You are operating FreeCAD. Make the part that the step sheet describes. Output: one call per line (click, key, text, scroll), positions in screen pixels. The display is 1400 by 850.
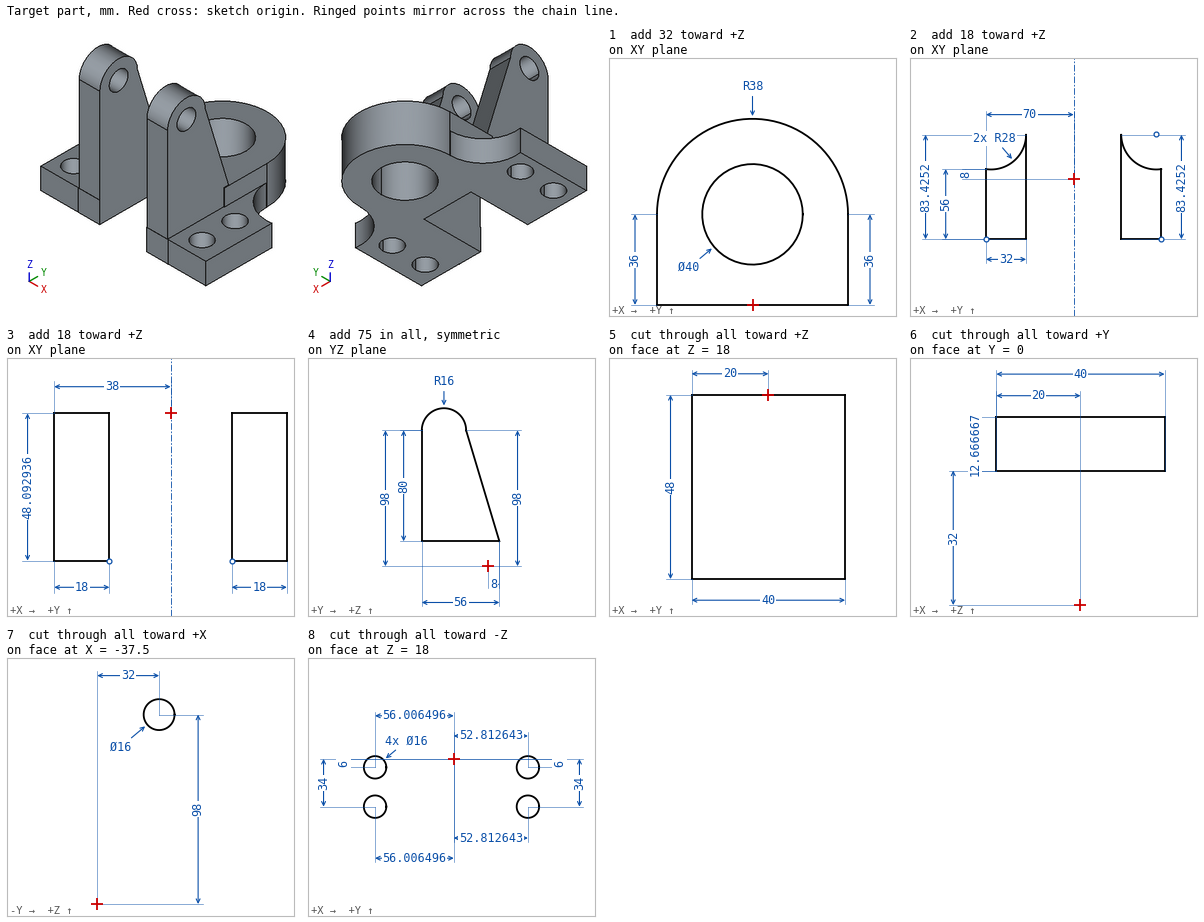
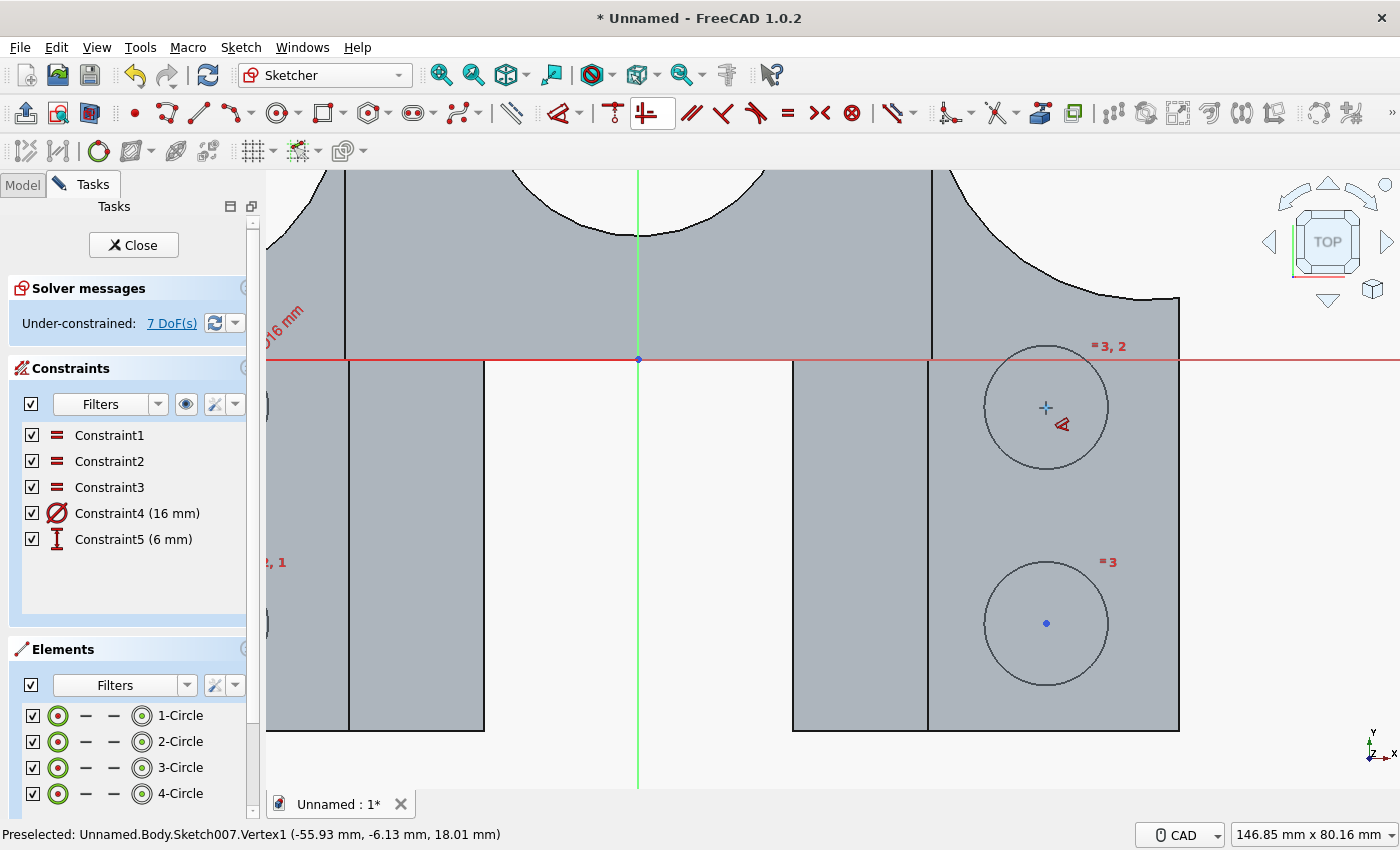
click(1046, 407)
click(1080, 384)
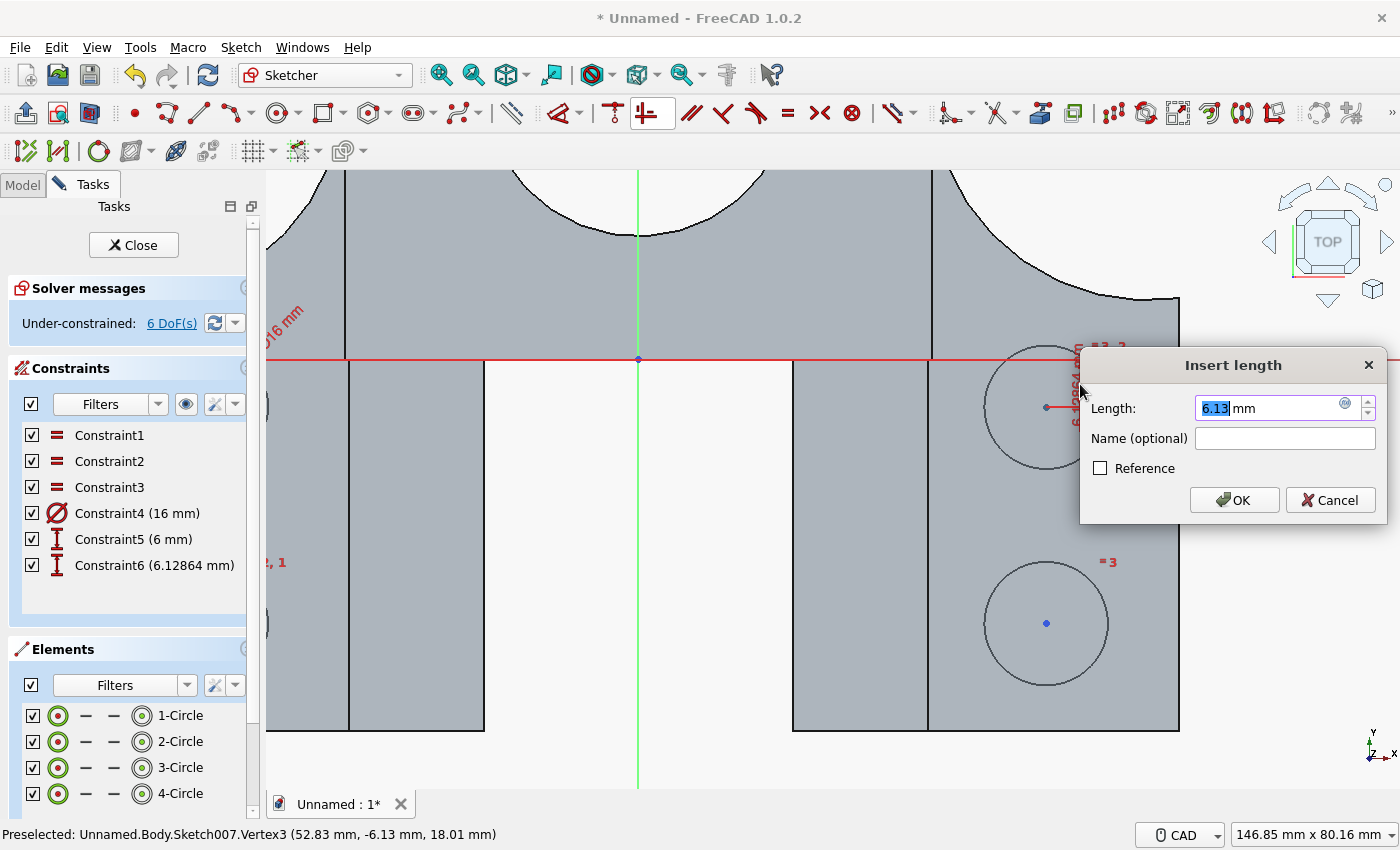
text(6)
key(Return)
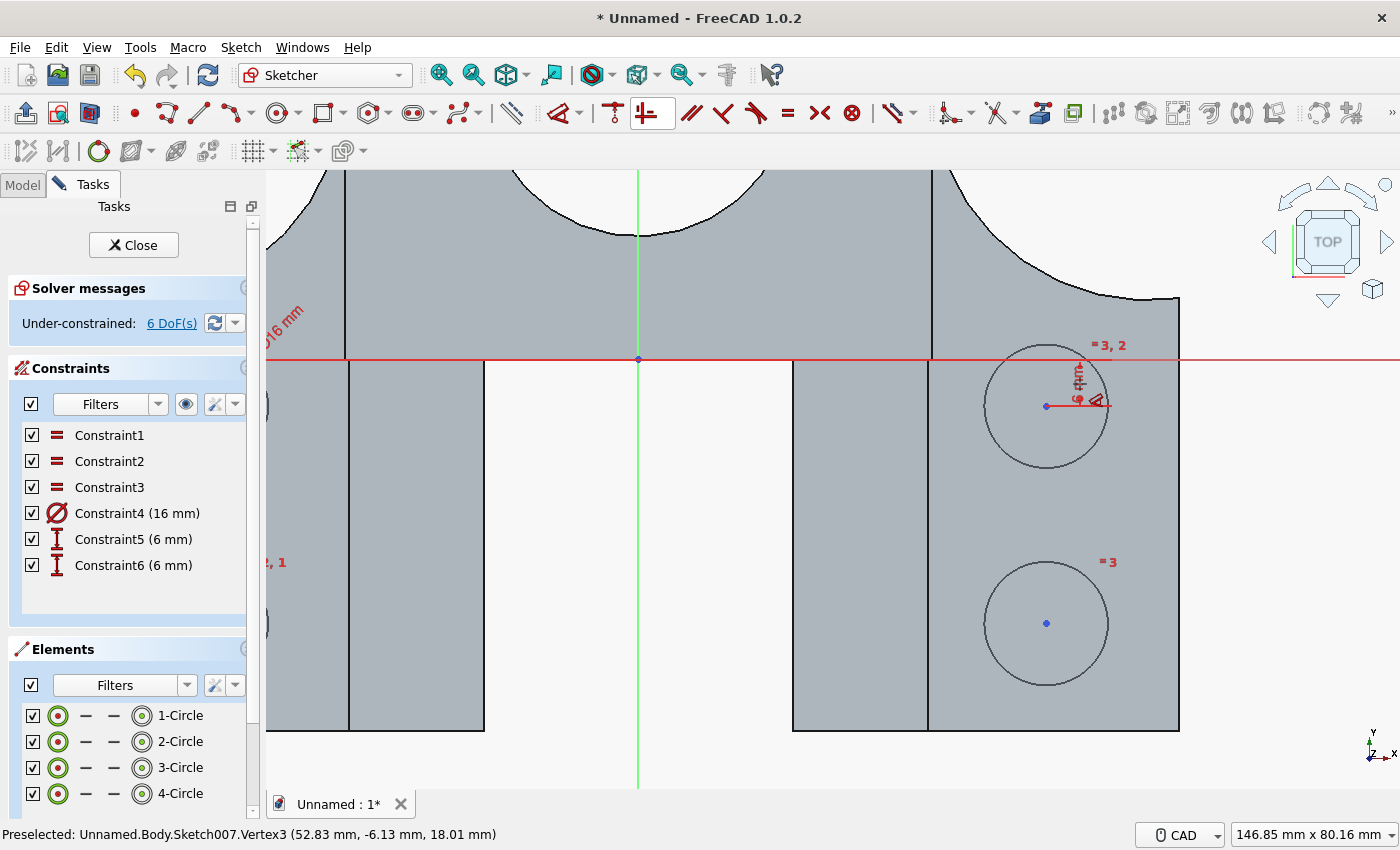
scroll(1046, 408, down, 2)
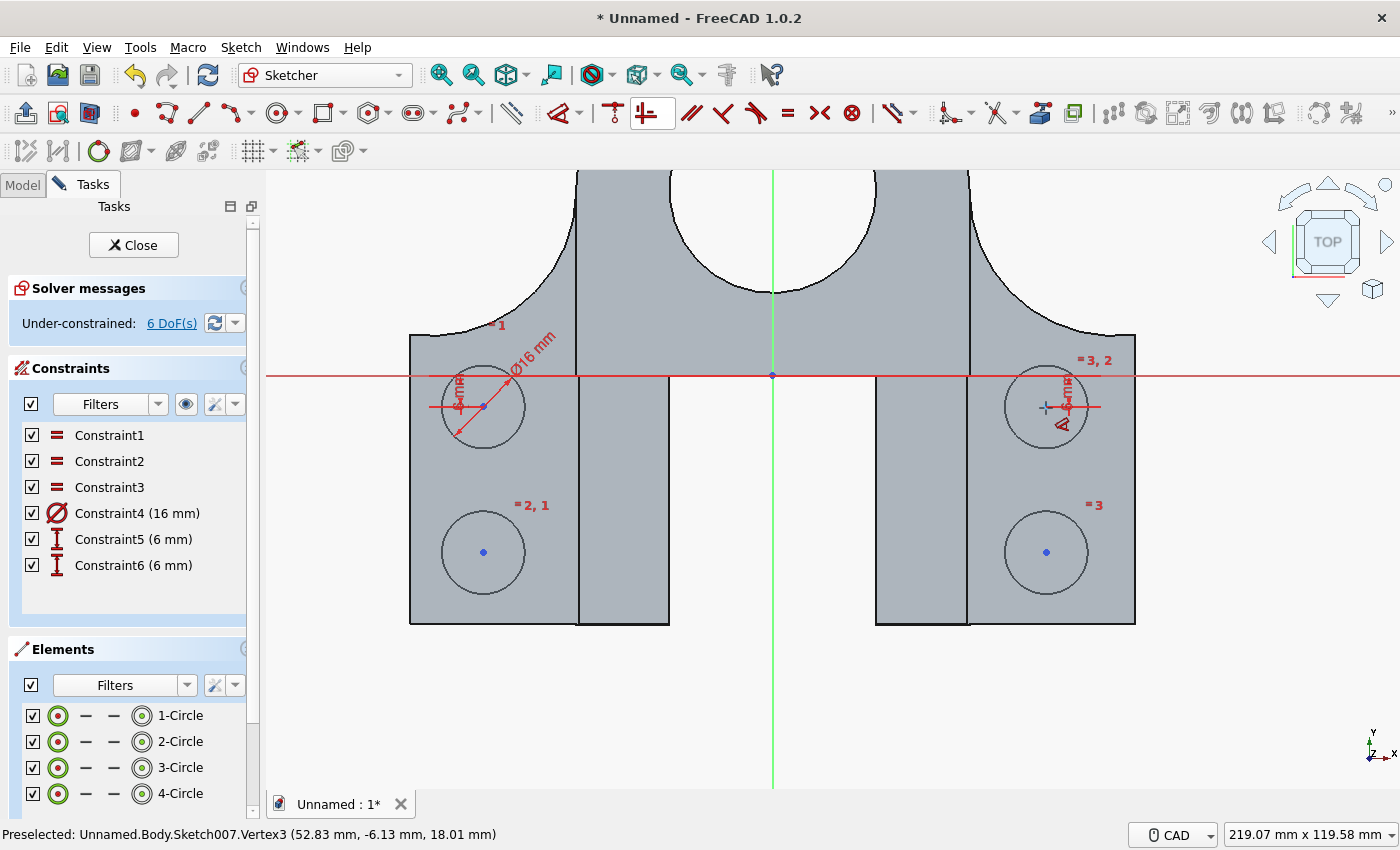
click(483, 553)
click(449, 464)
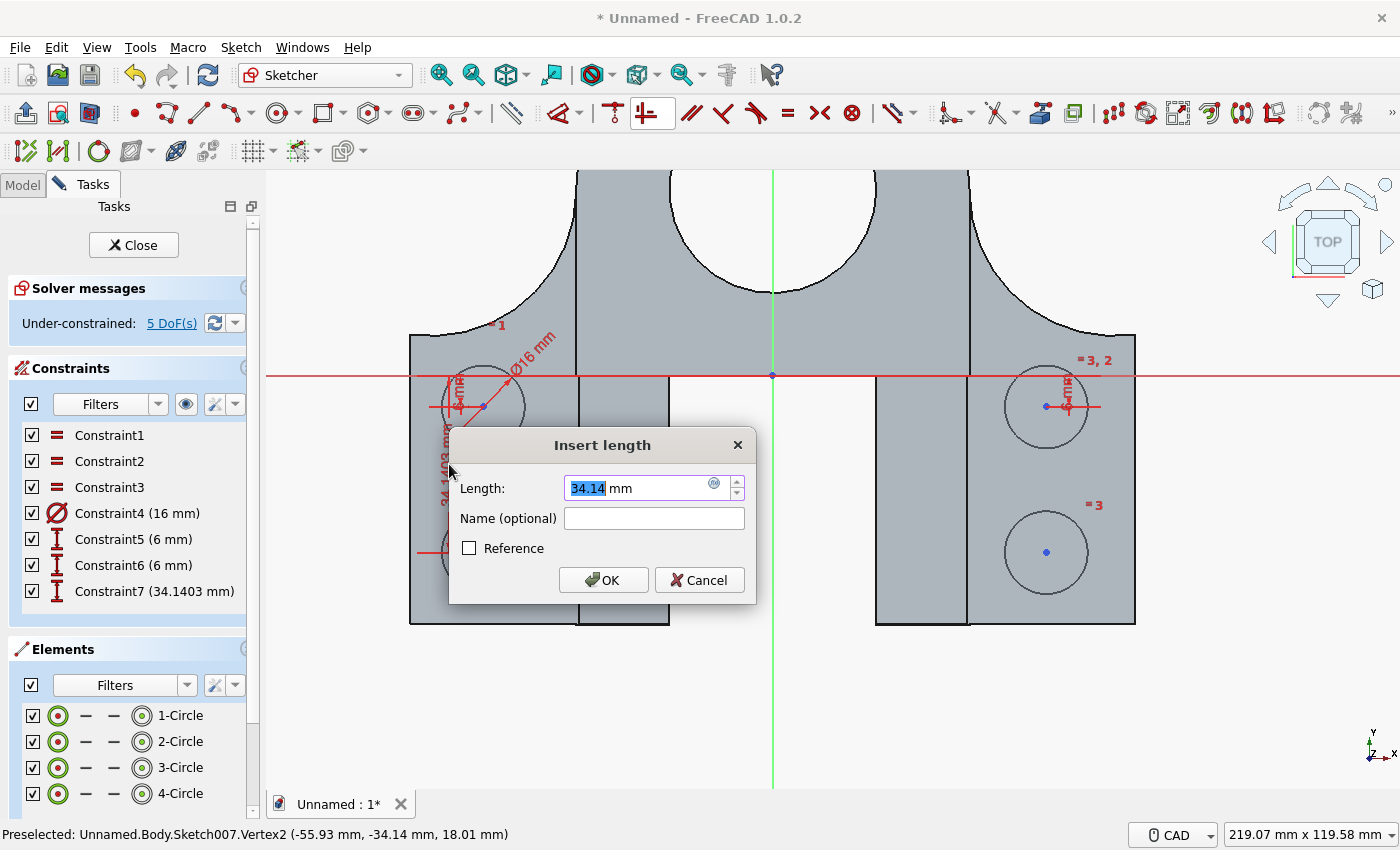
text(34)
key(Return)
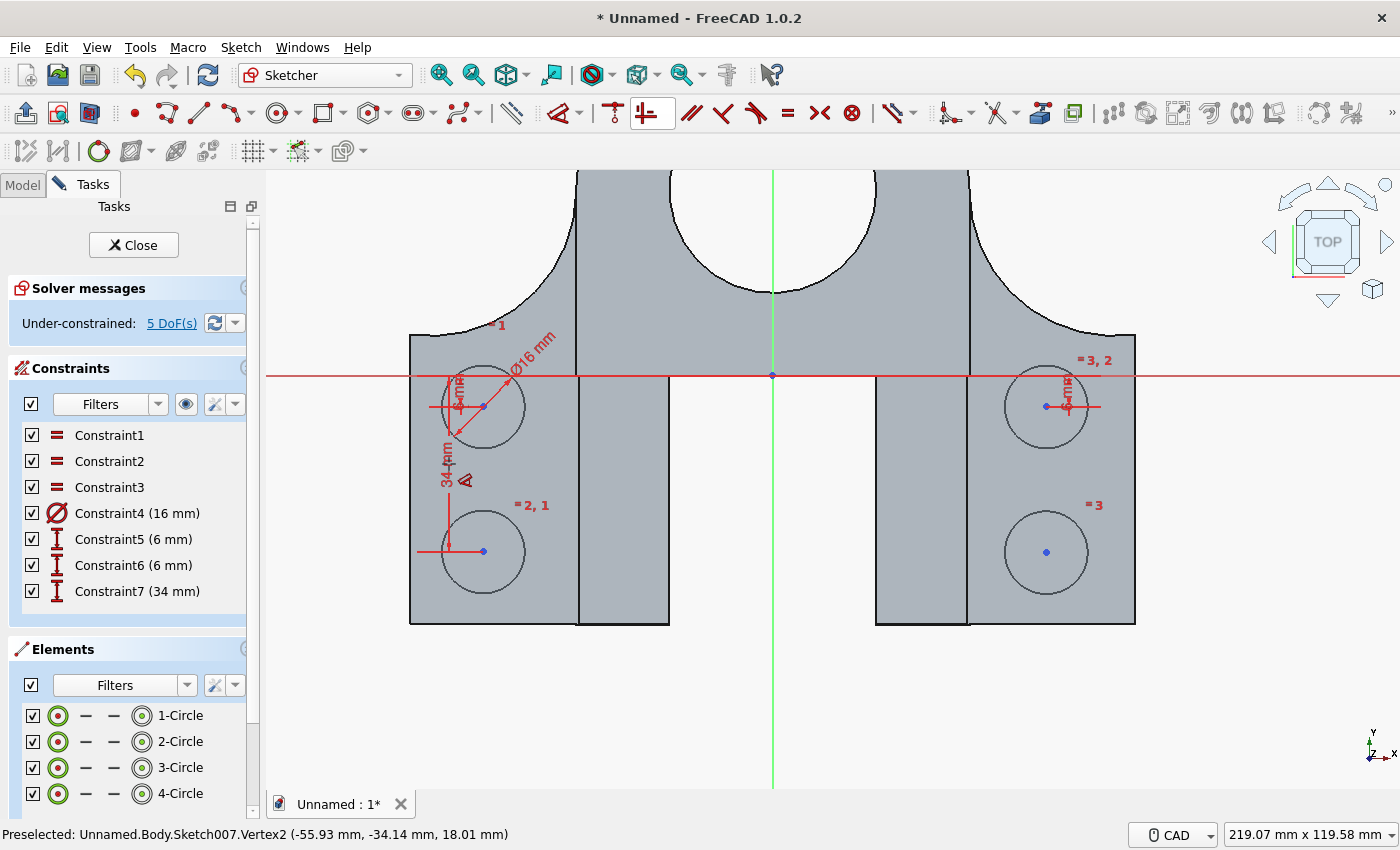
click(1046, 553)
click(1080, 464)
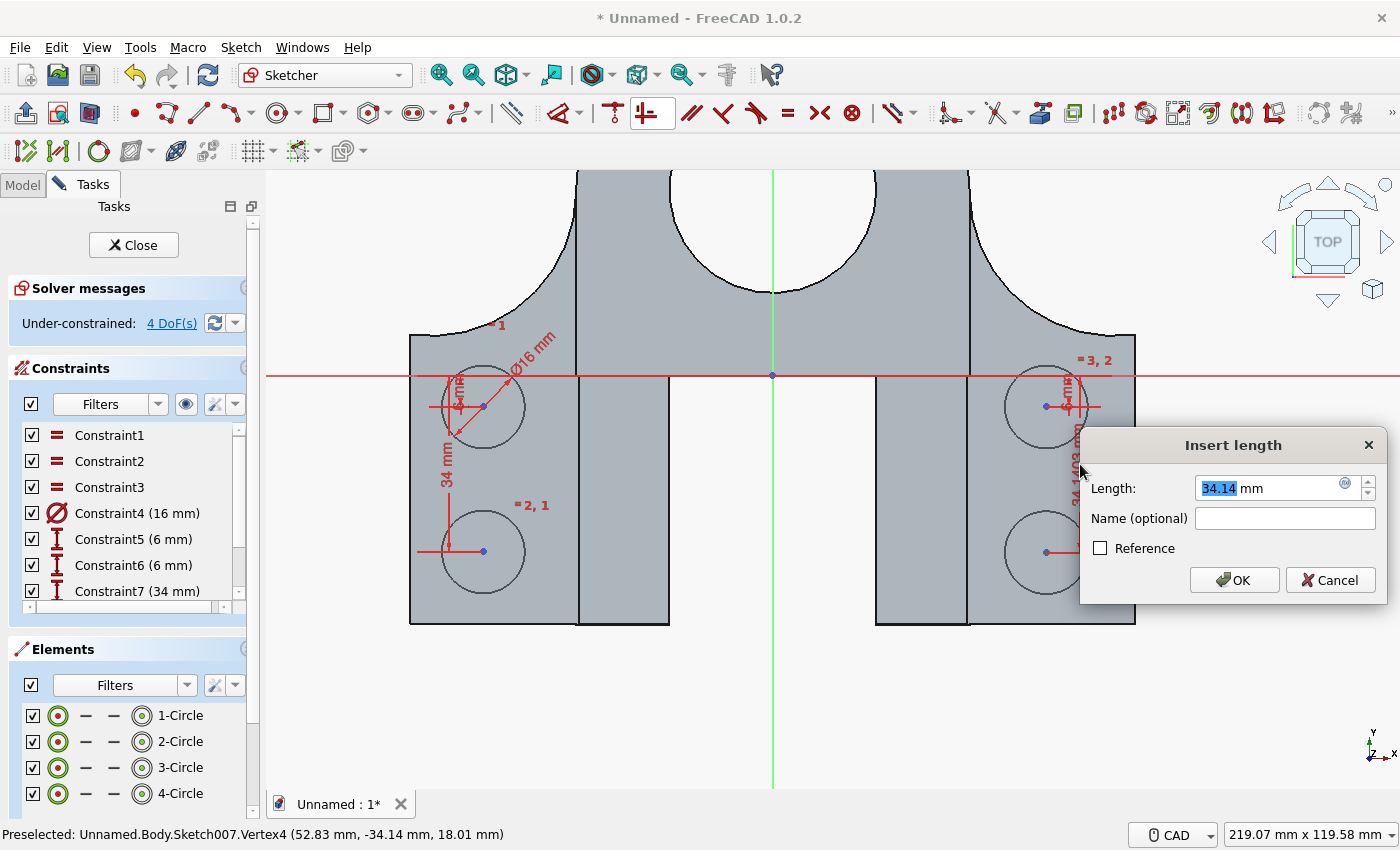
text(34)
key(Return)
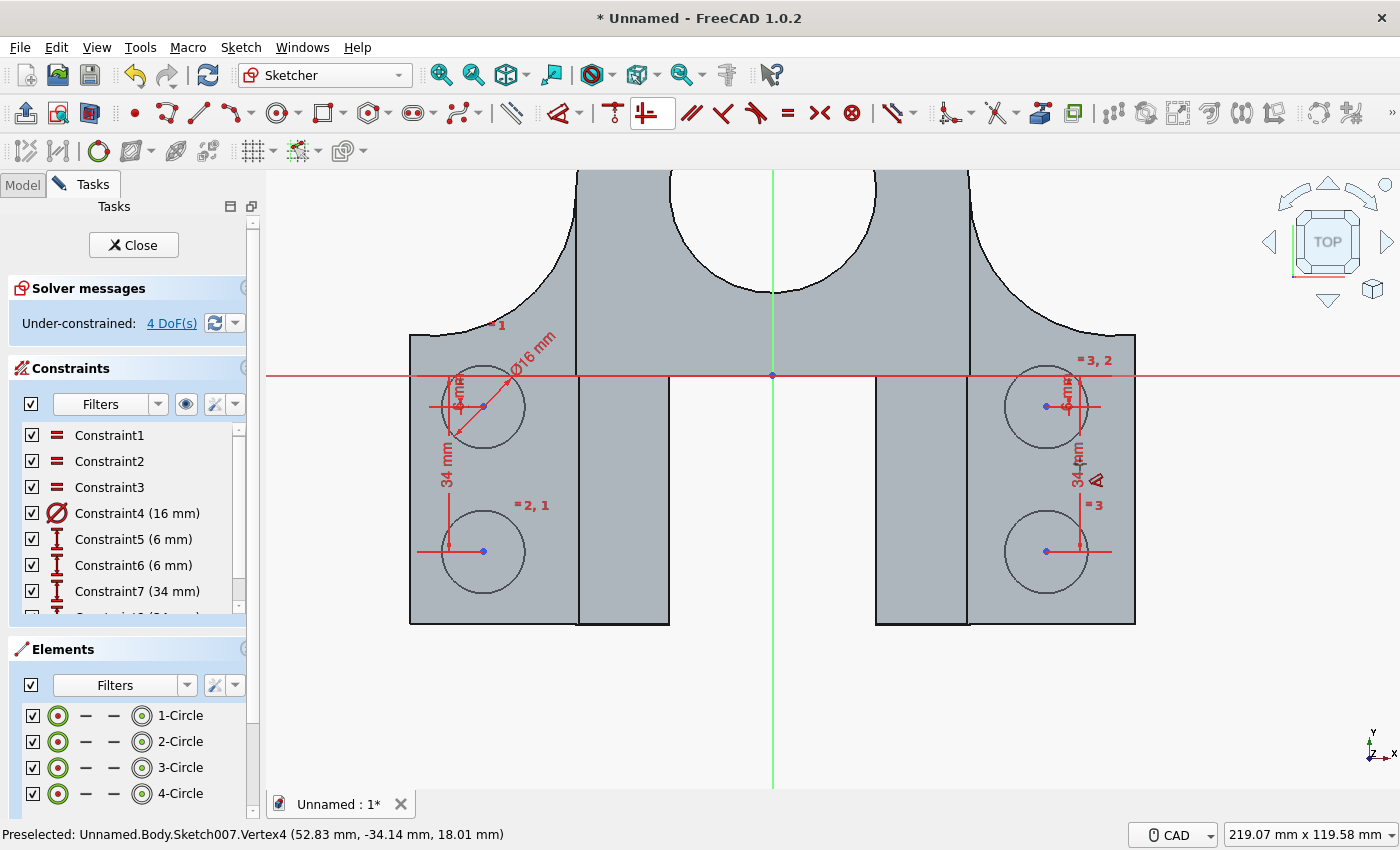
click(483, 407)
click(628, 342)